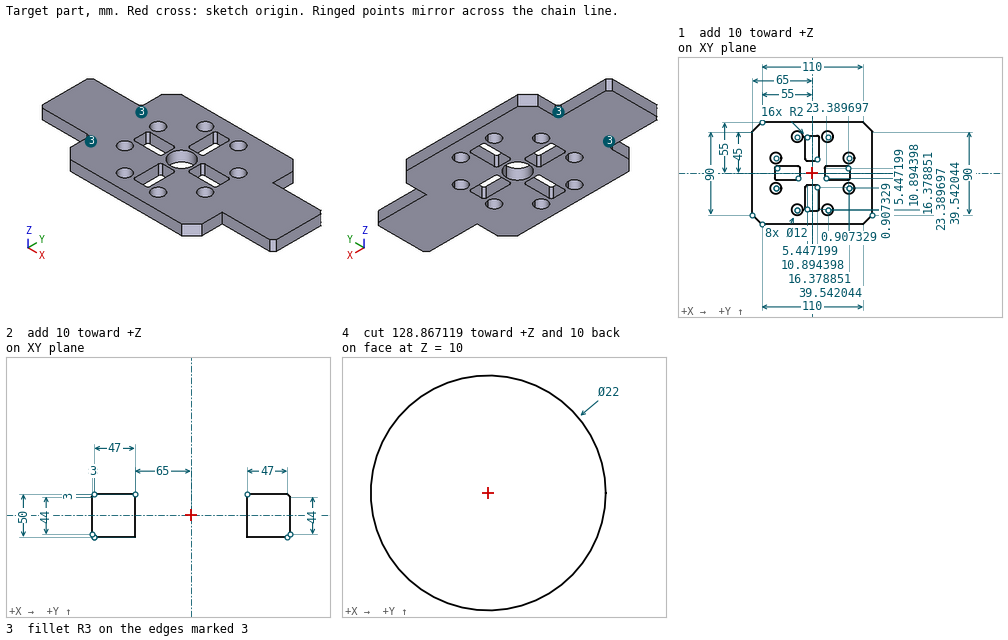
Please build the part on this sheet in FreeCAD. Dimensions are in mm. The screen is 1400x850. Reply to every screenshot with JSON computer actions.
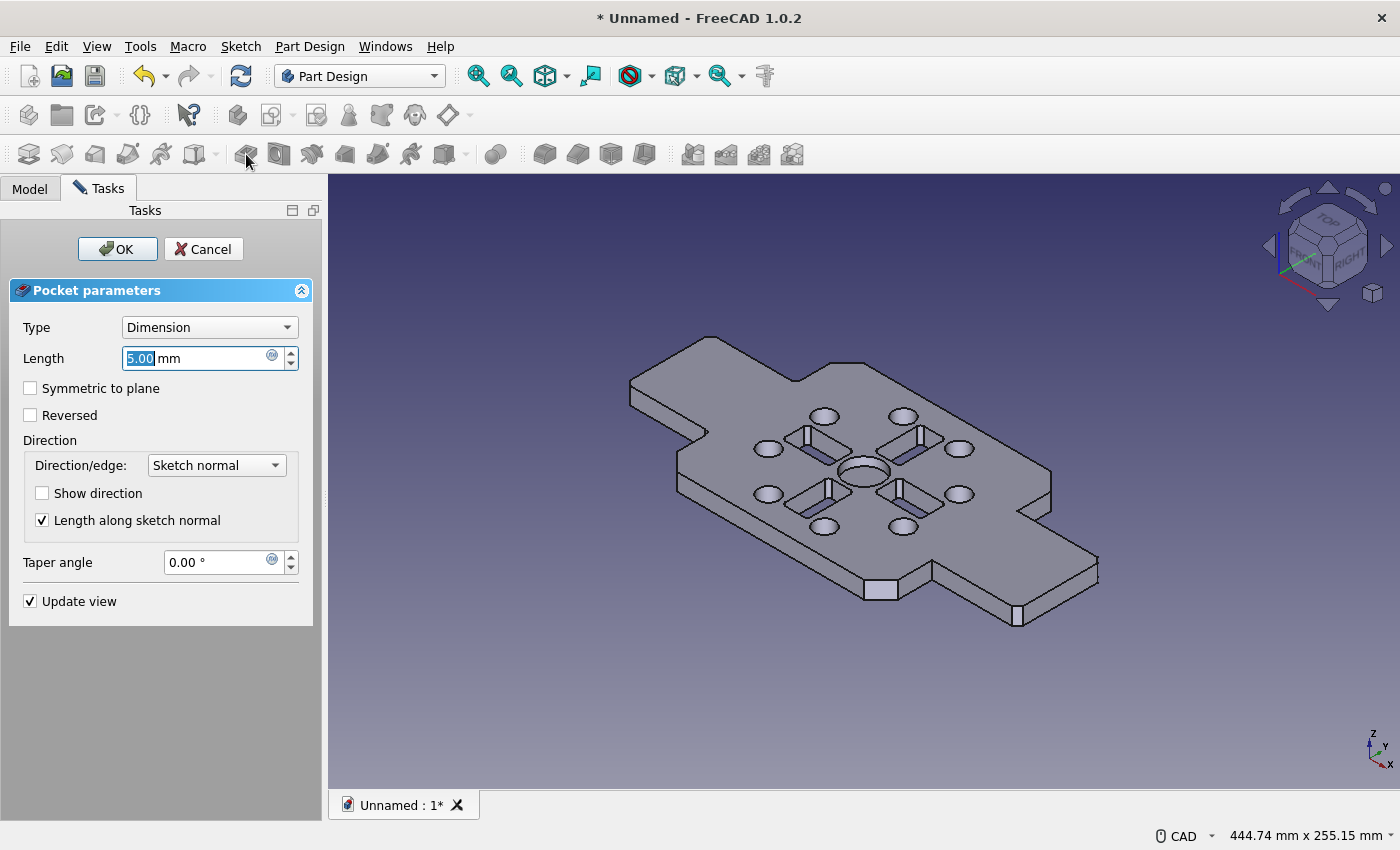
{"action": "left_click", "coordinate": [210, 328]}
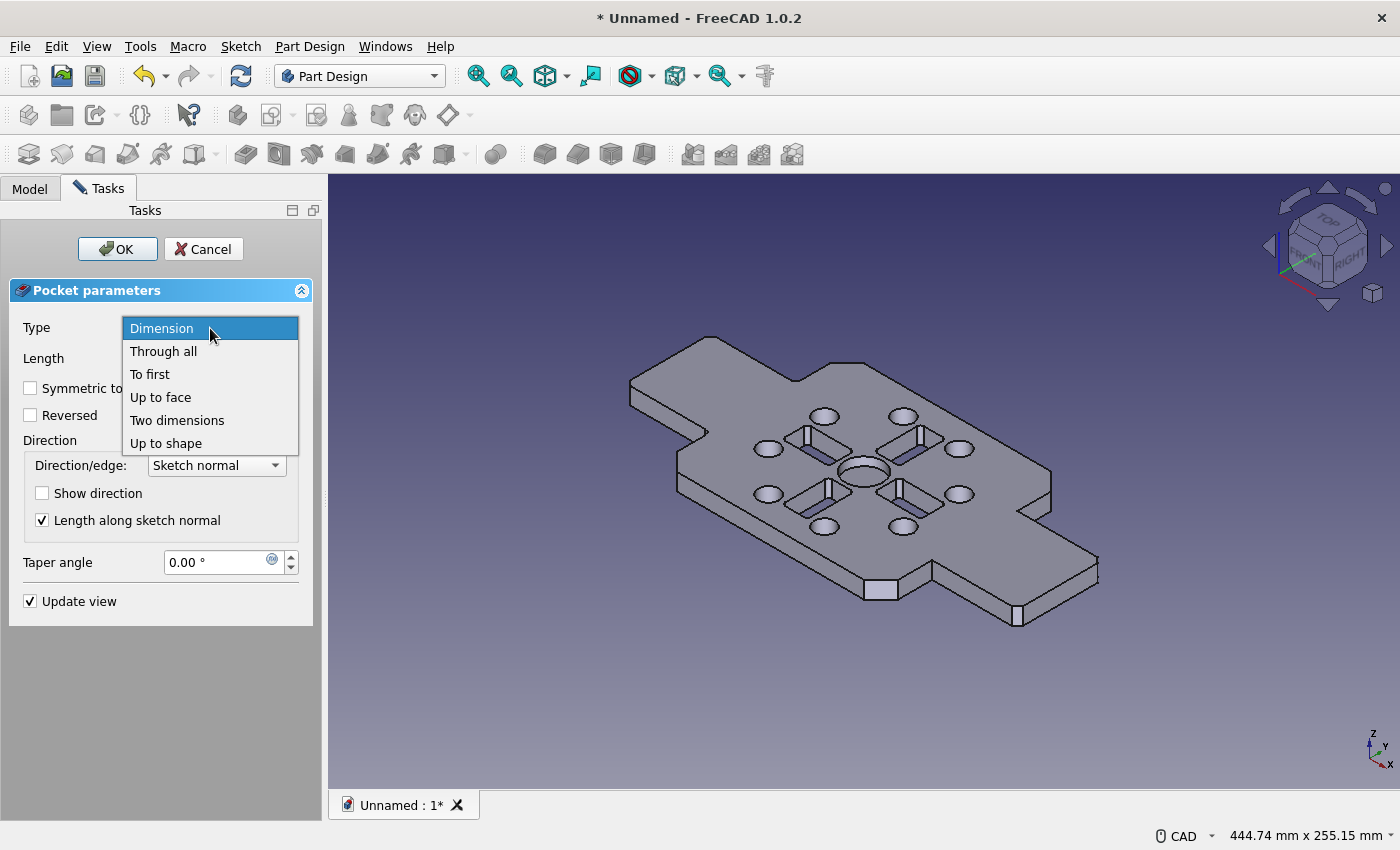
{"action": "left_click", "coordinate": [208, 420]}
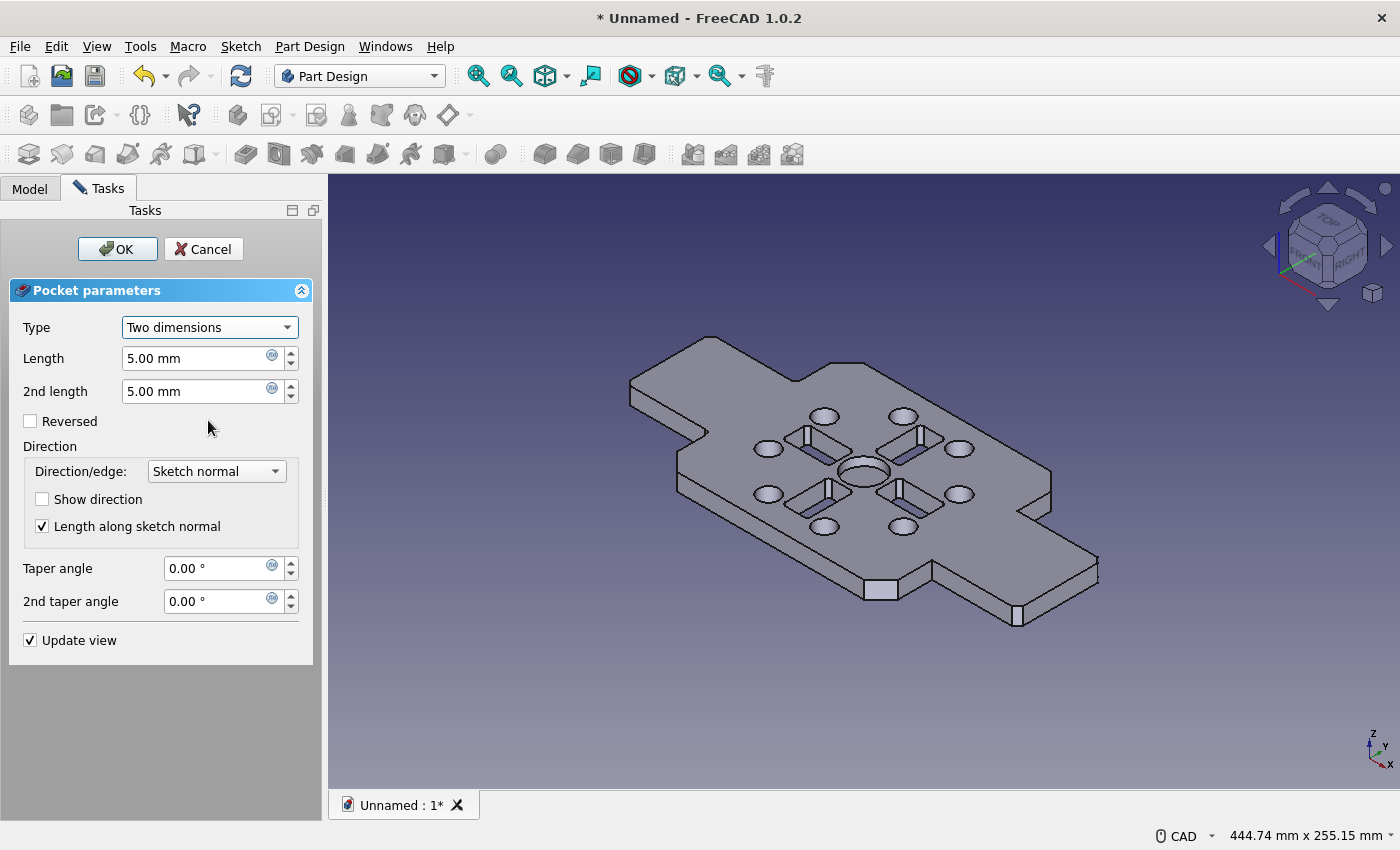
{"action": "triple_click", "coordinate": [204, 358]}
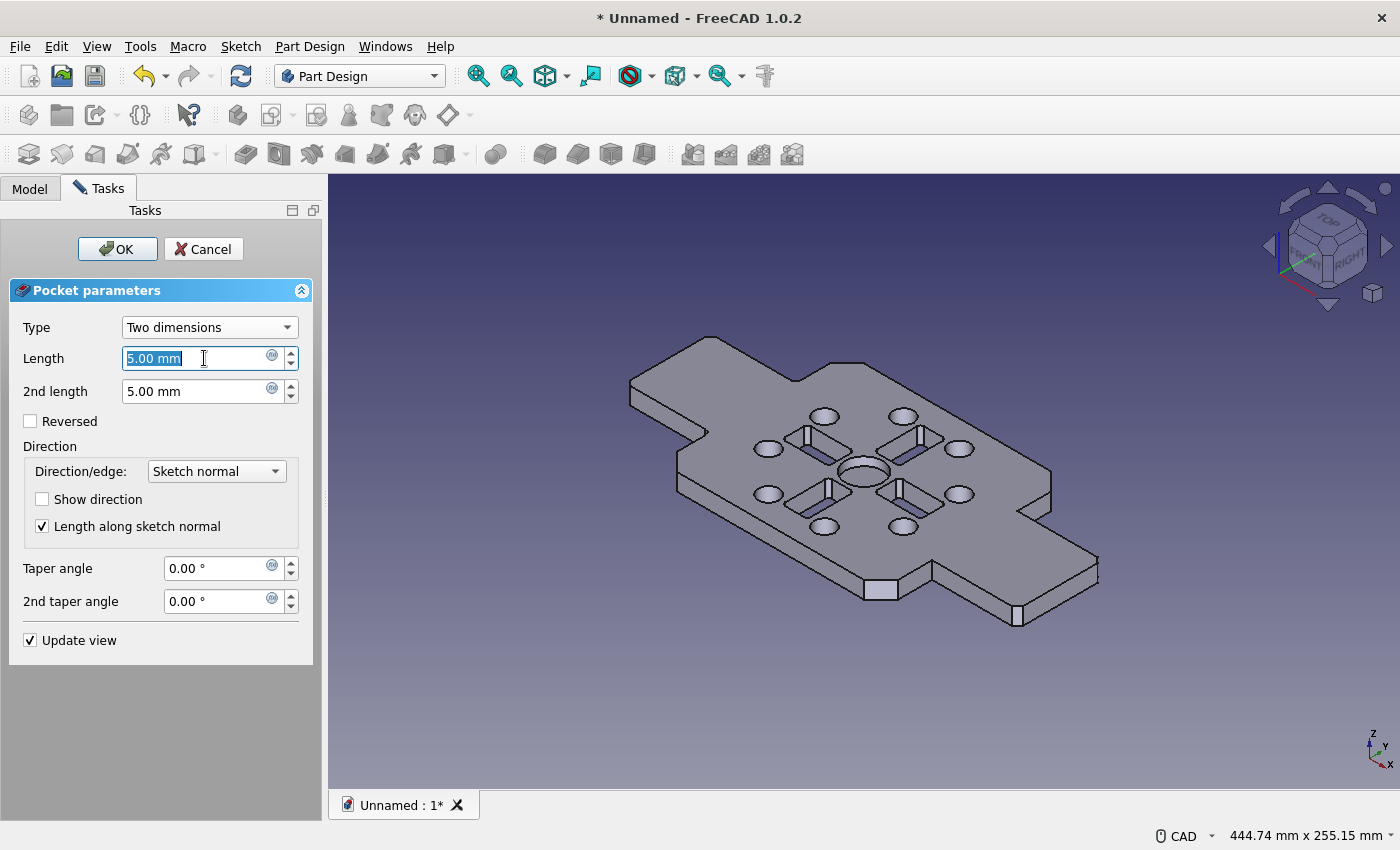
{"action": "type", "text": "128.867119"}
{"action": "key", "text": "Tab"}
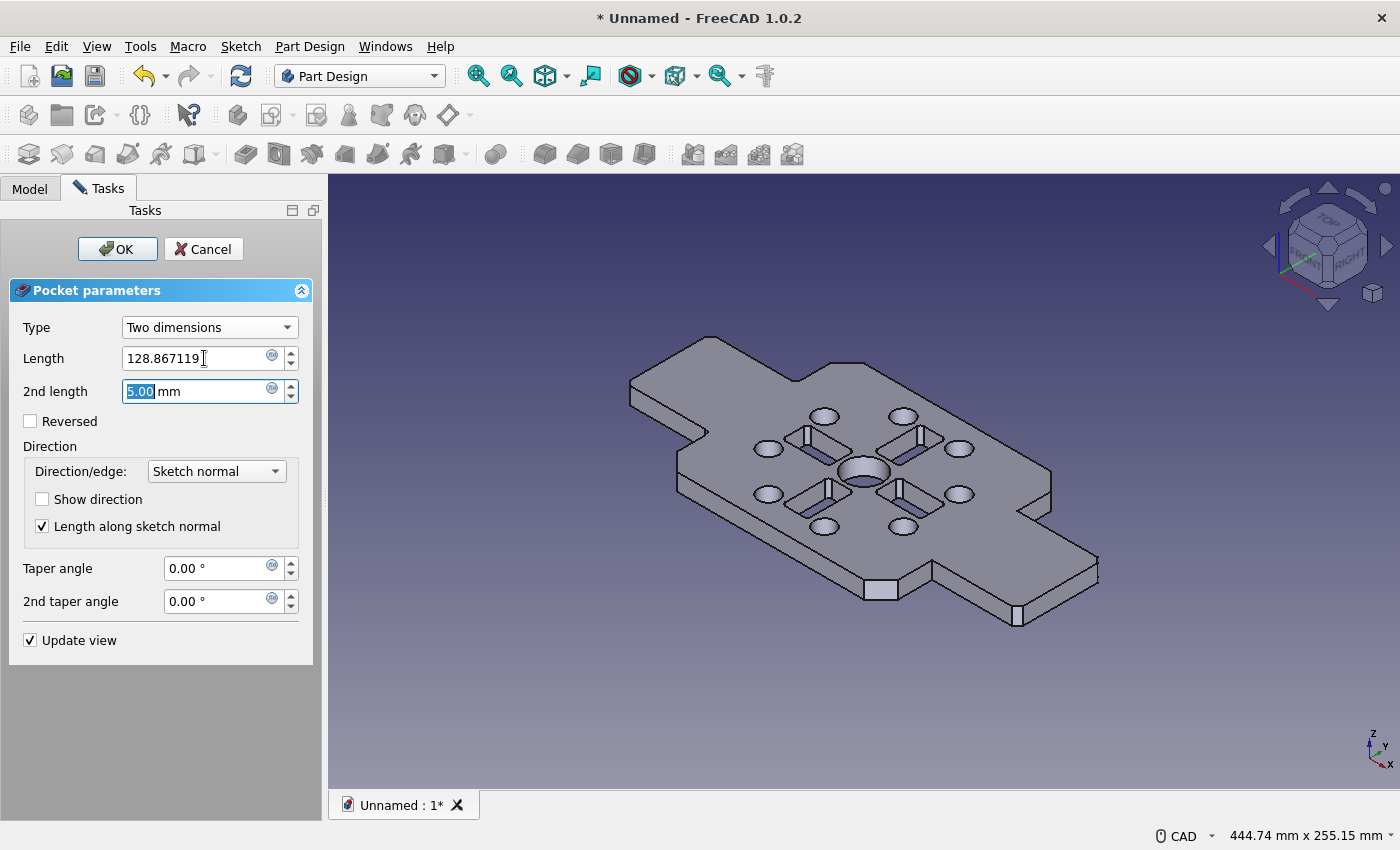
{"action": "type", "text": "10"}
{"action": "key", "text": "Tab"}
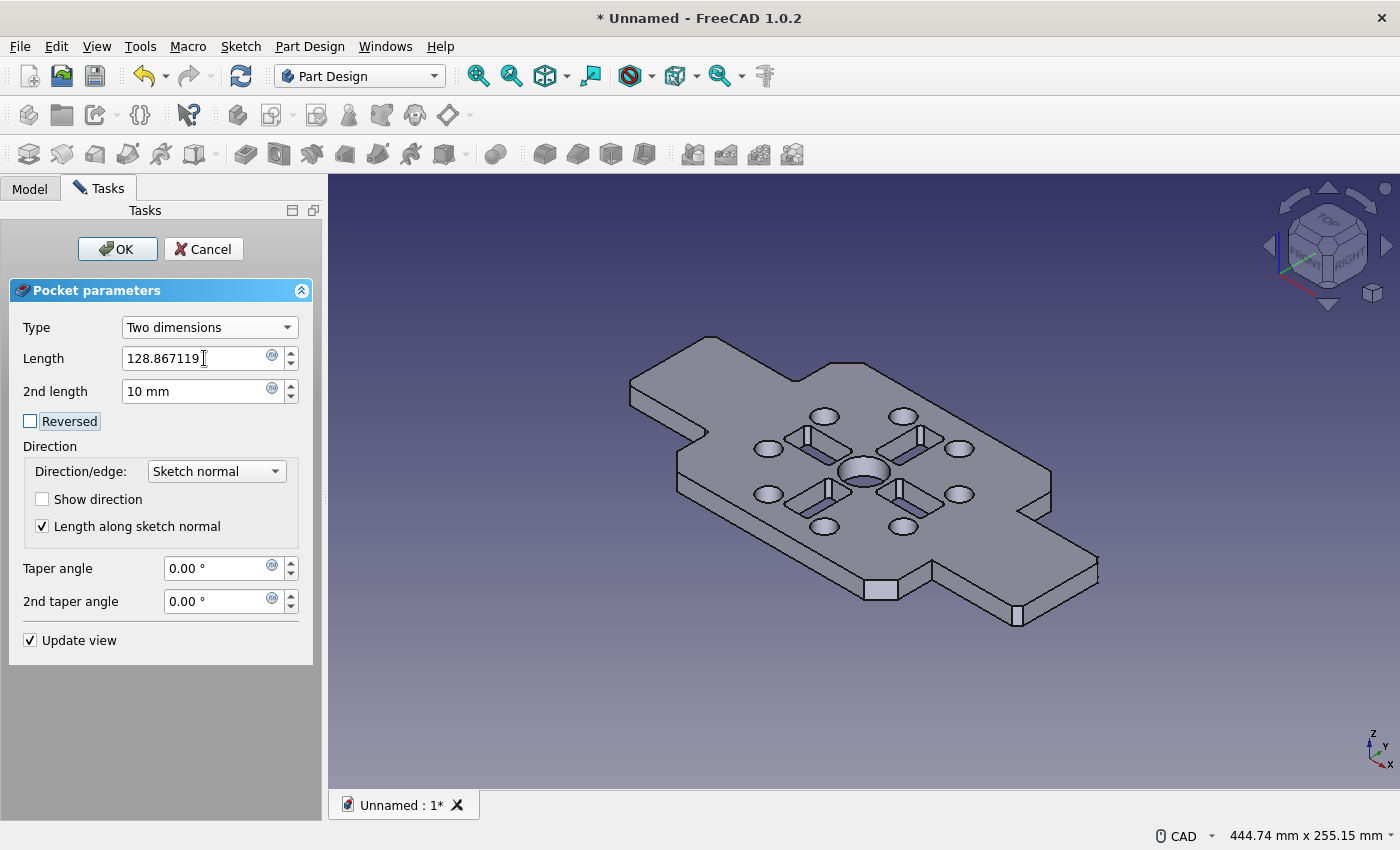
{"action": "left_click", "coordinate": [31, 421]}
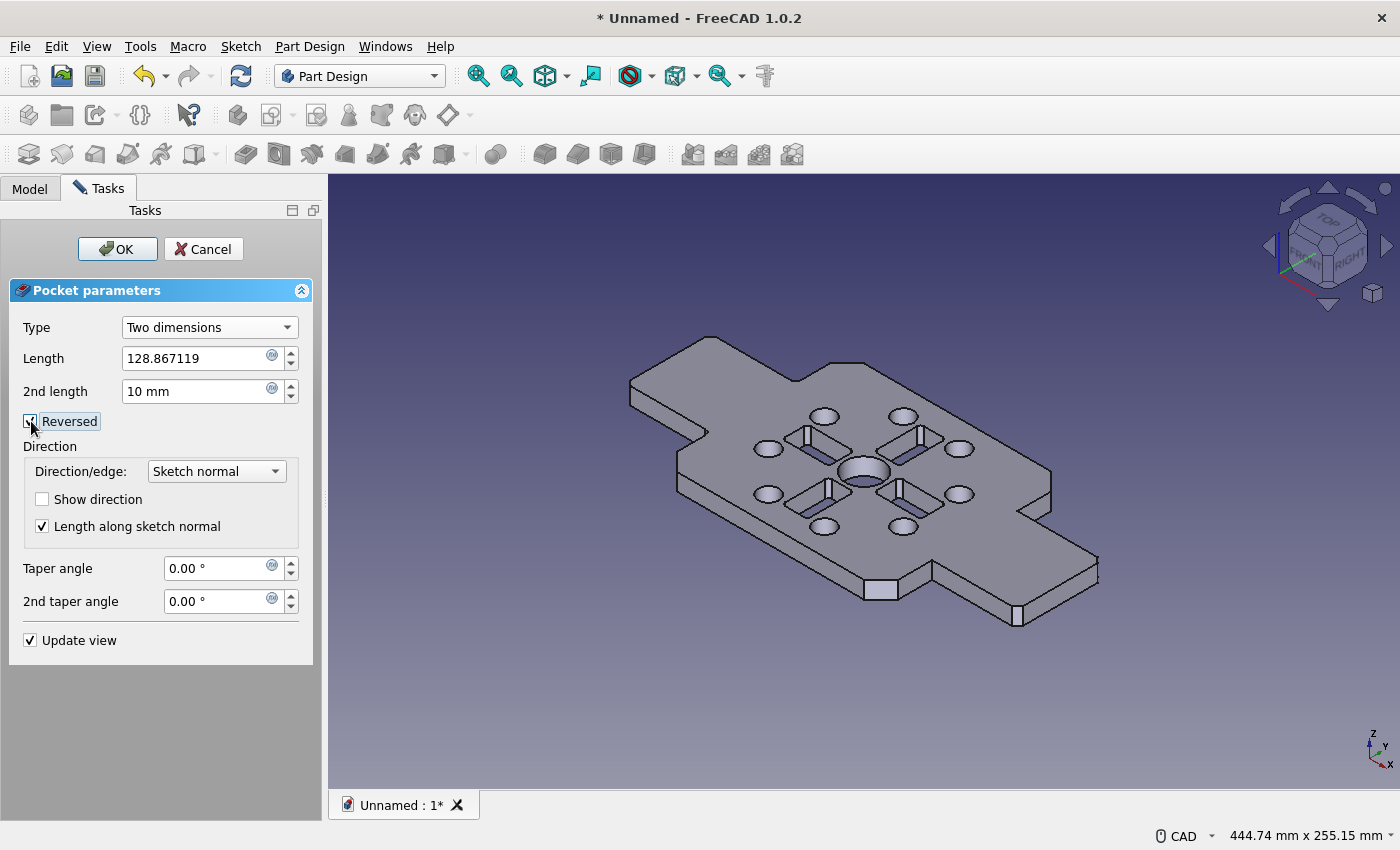
{"action": "left_click", "coordinate": [118, 249]}